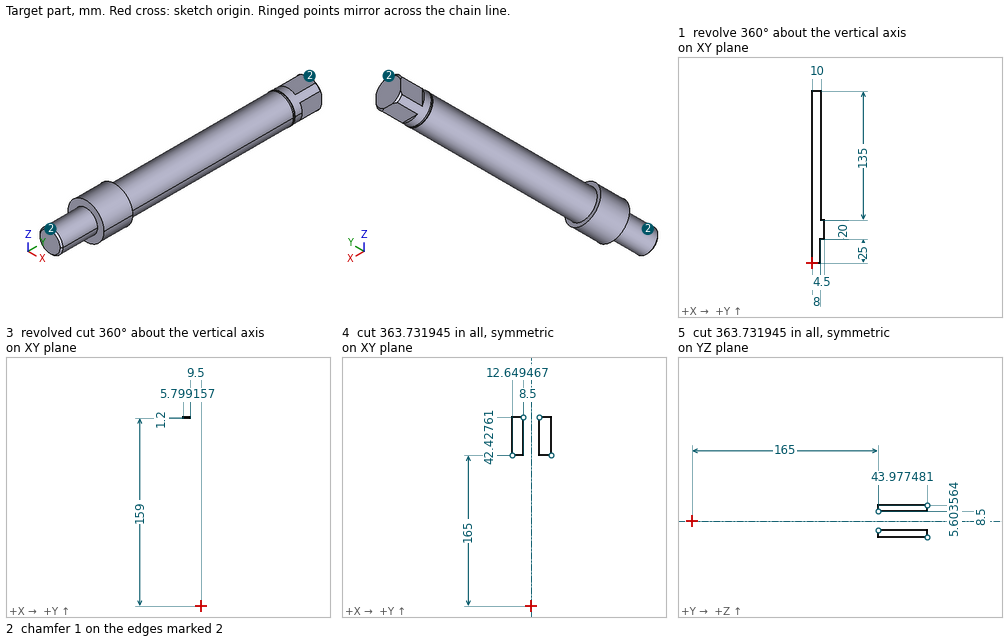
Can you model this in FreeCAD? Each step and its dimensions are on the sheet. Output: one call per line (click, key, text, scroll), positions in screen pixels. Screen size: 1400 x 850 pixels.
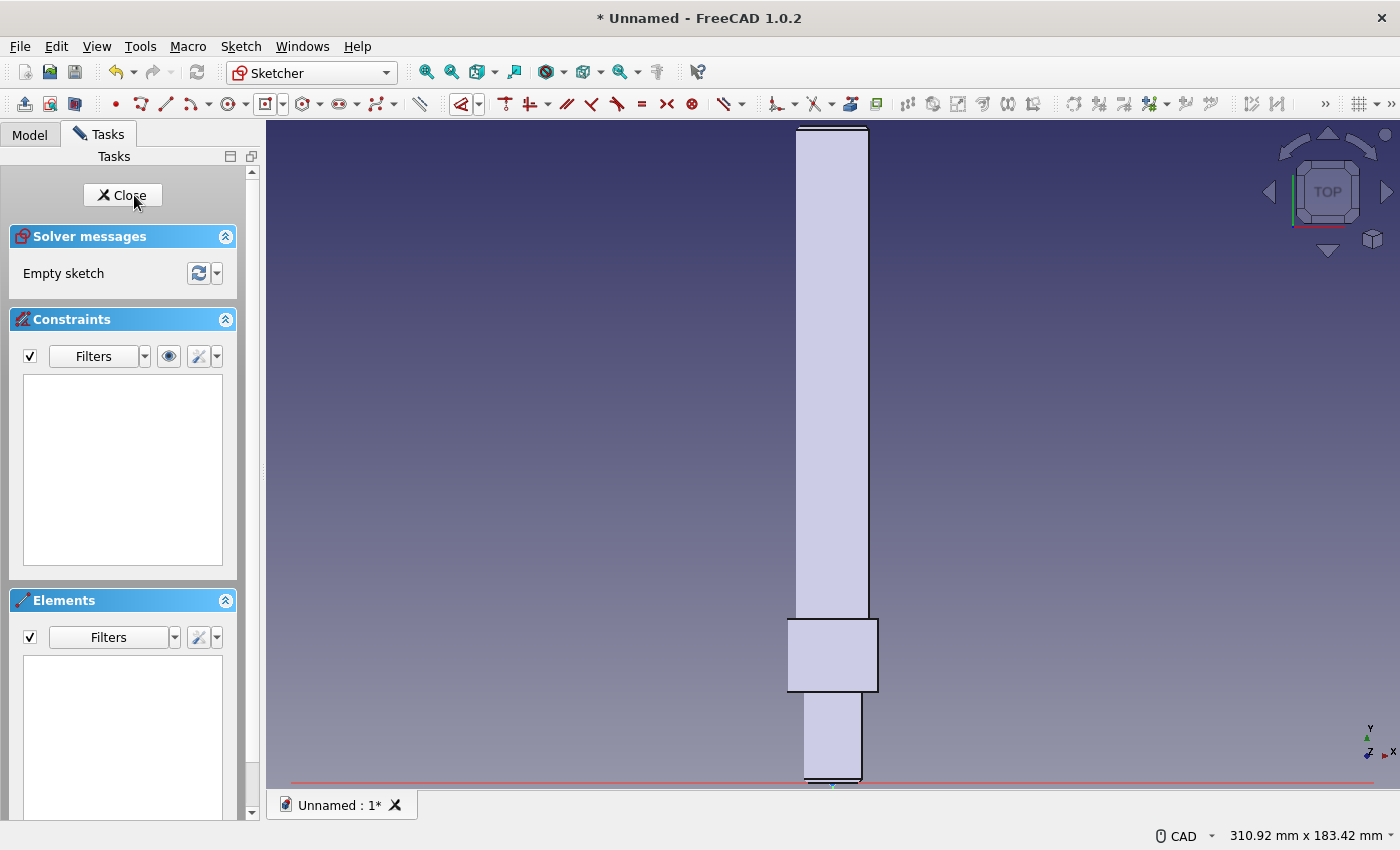
key(q)
key(s)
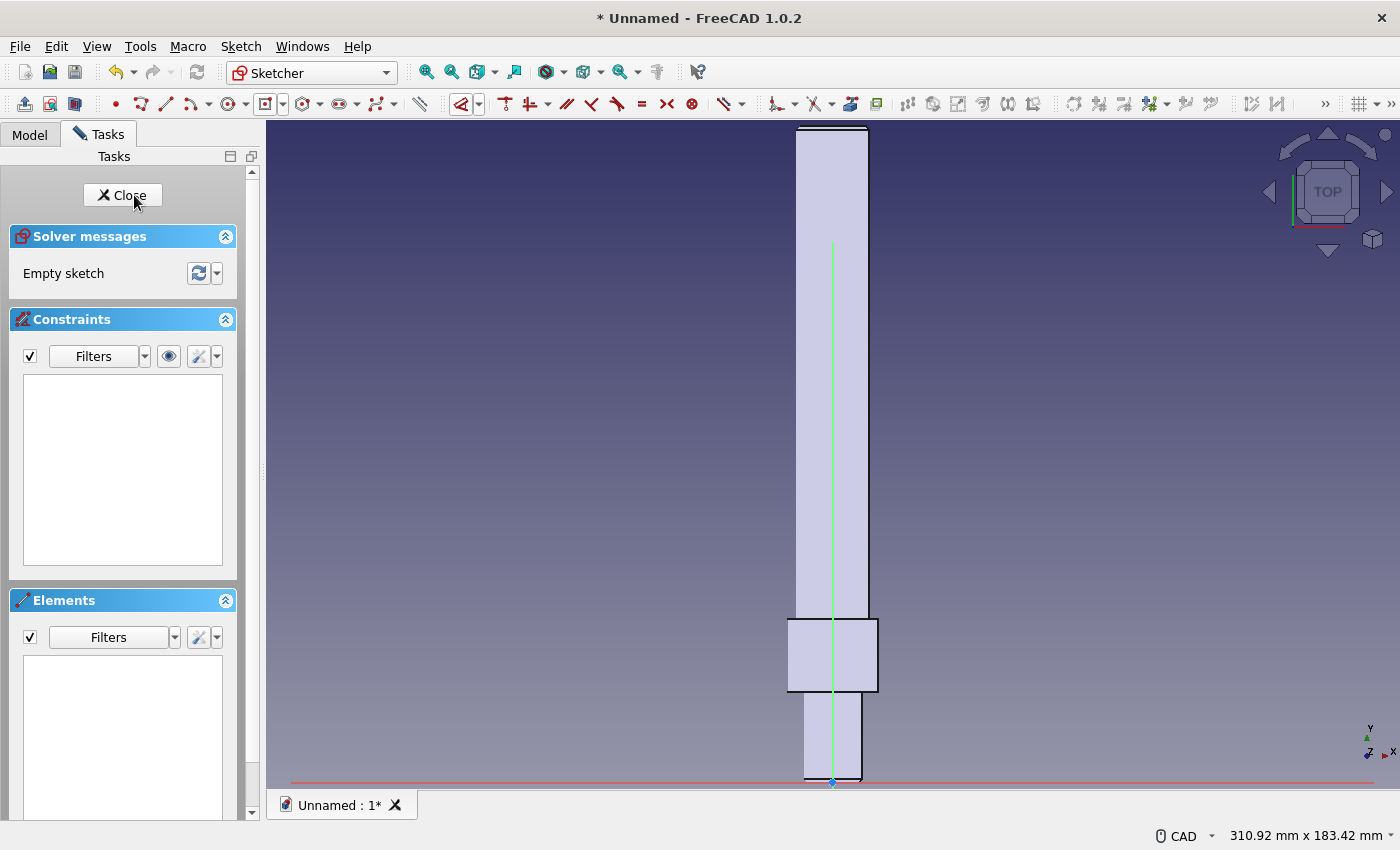
scroll(789, 187, up, 15)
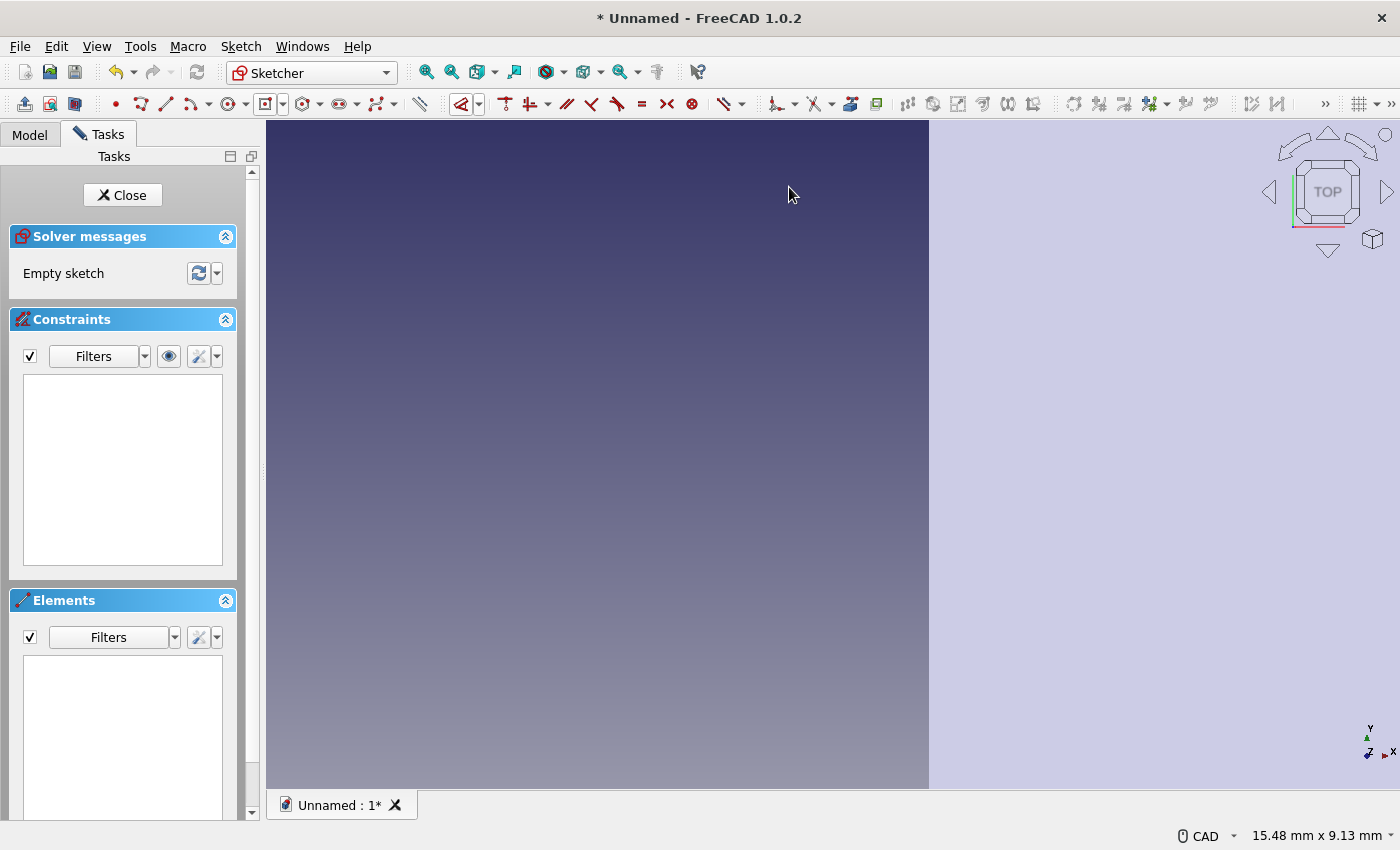
scroll(729, 469, up, 2)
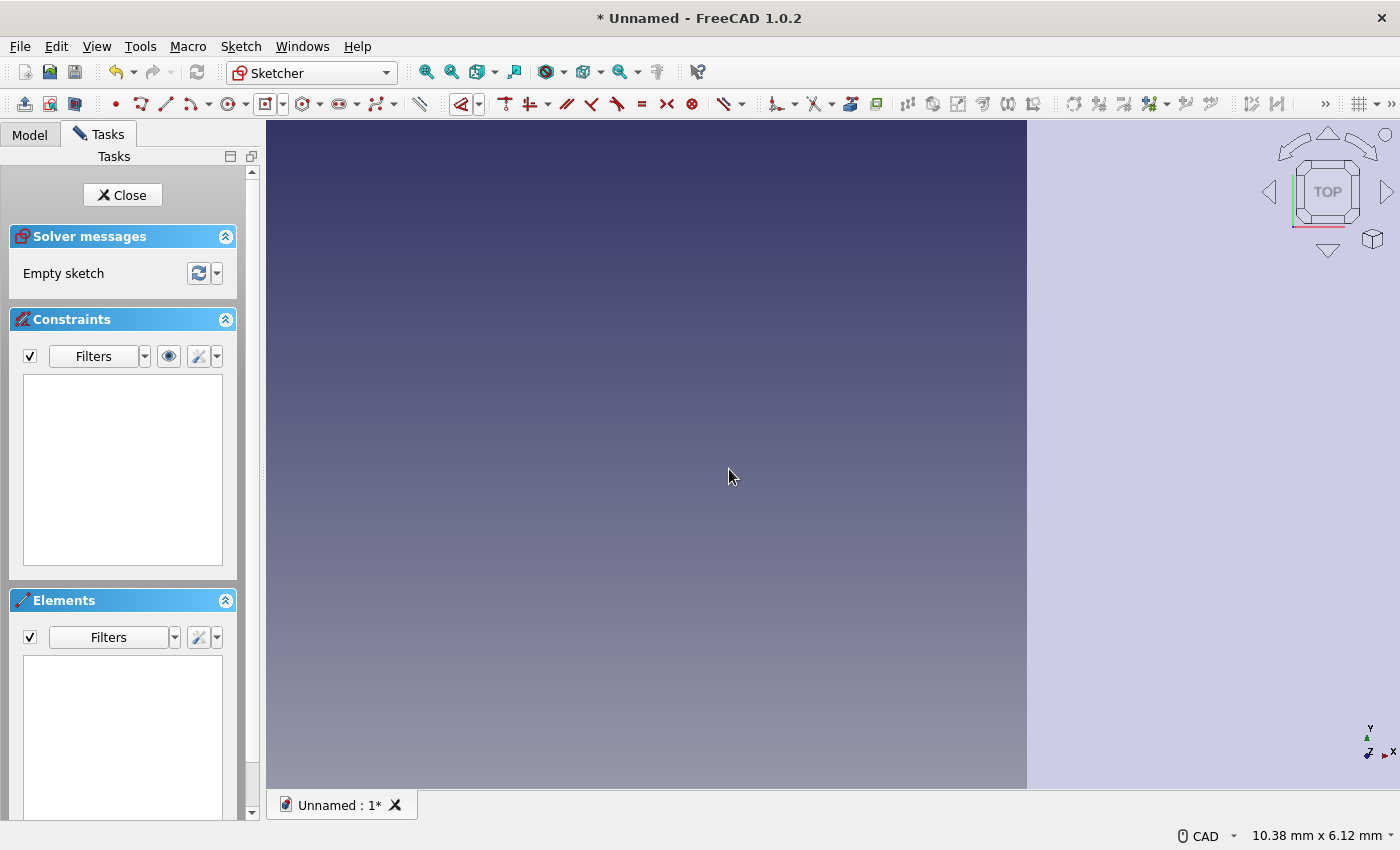
click(282, 104)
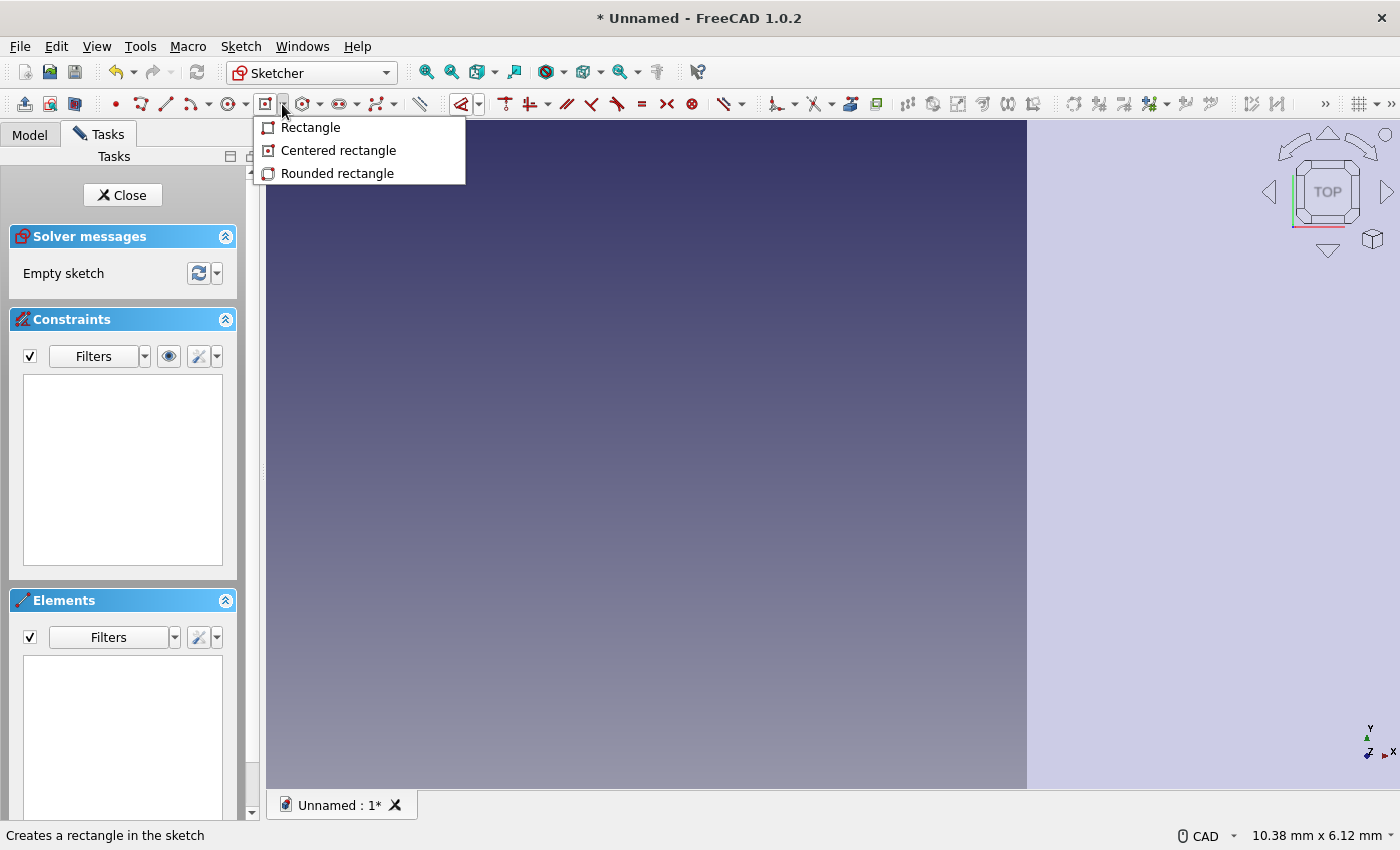
click(360, 128)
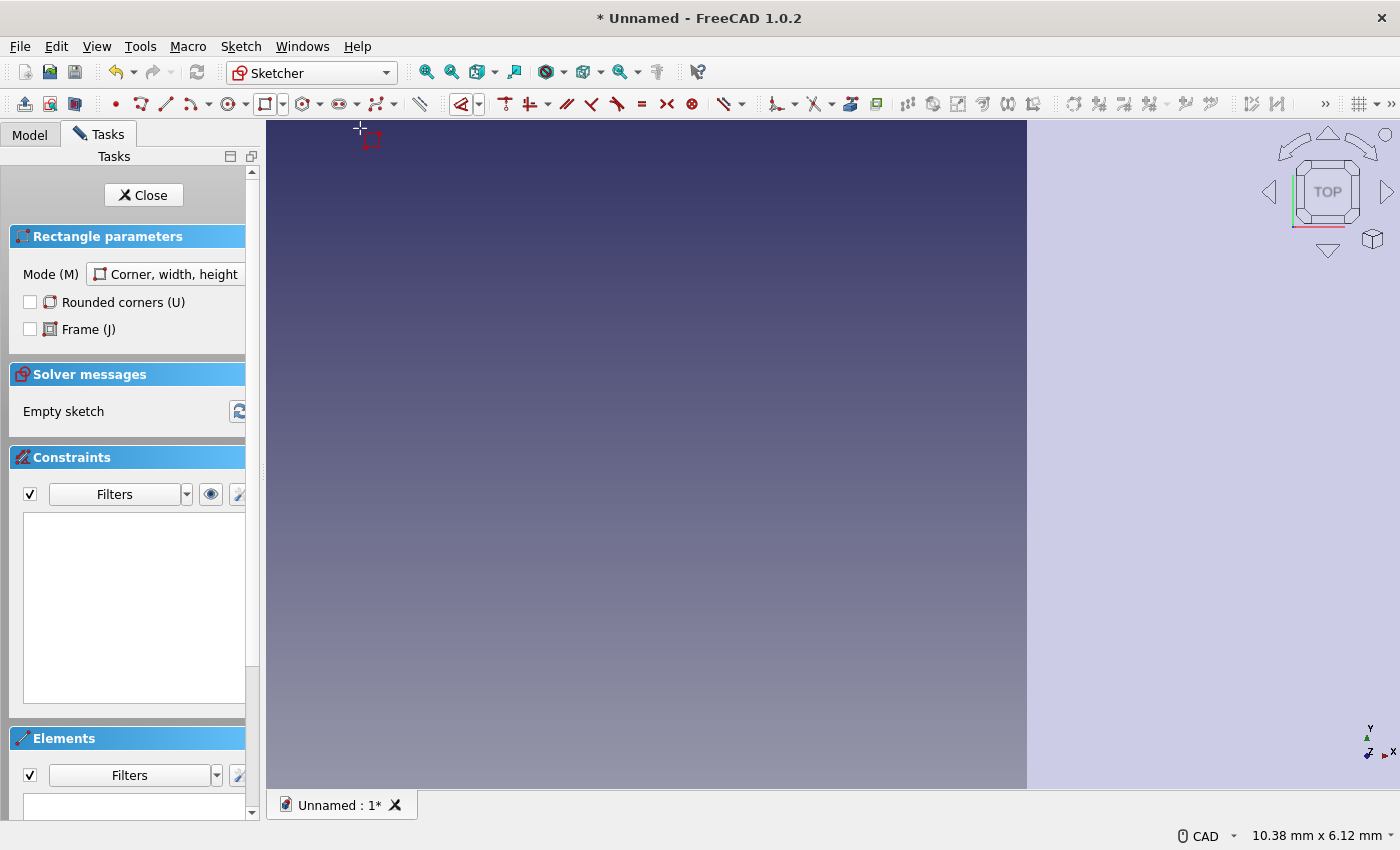
click(448, 389)
click(1081, 520)
key(Escape)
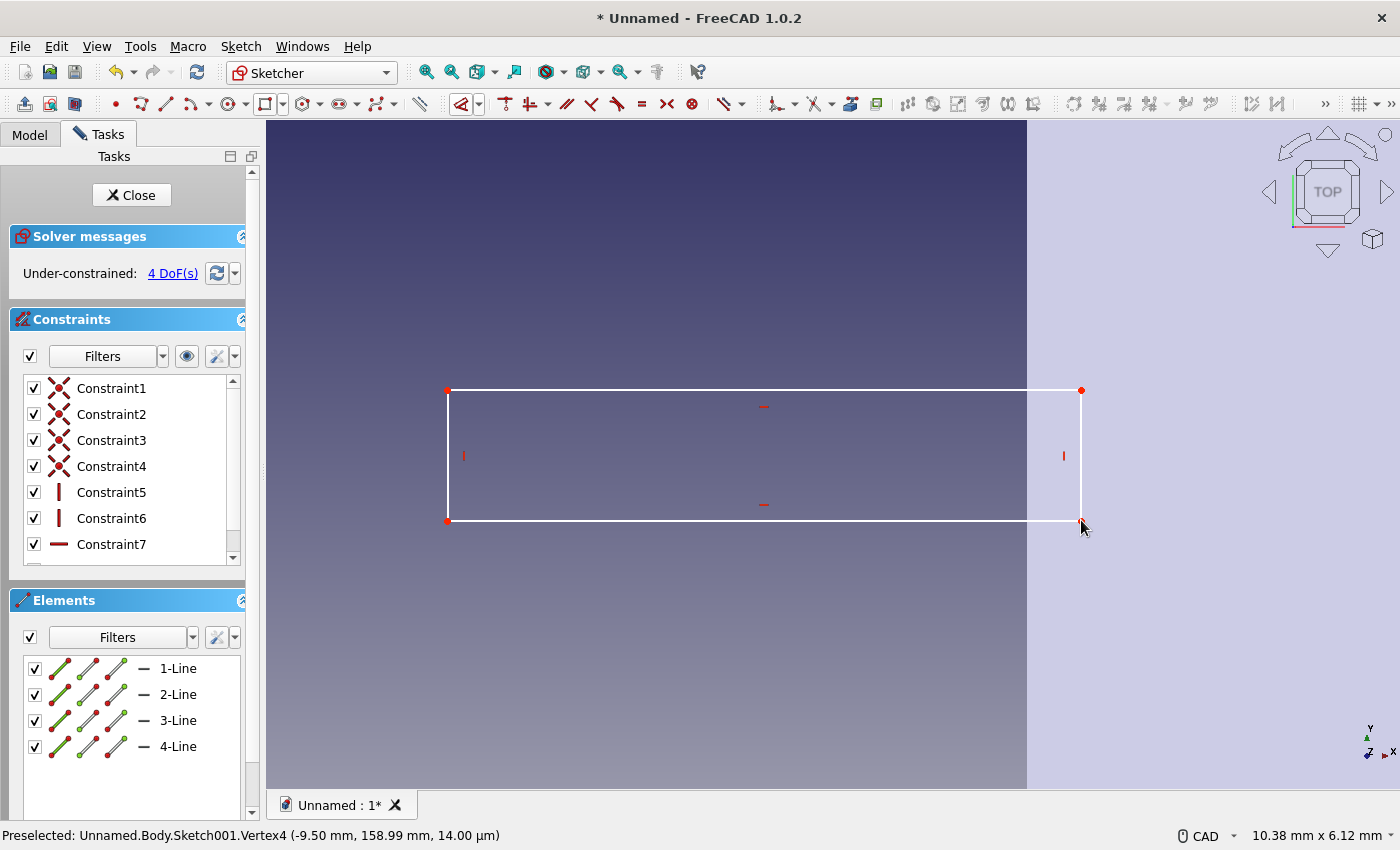
click(460, 104)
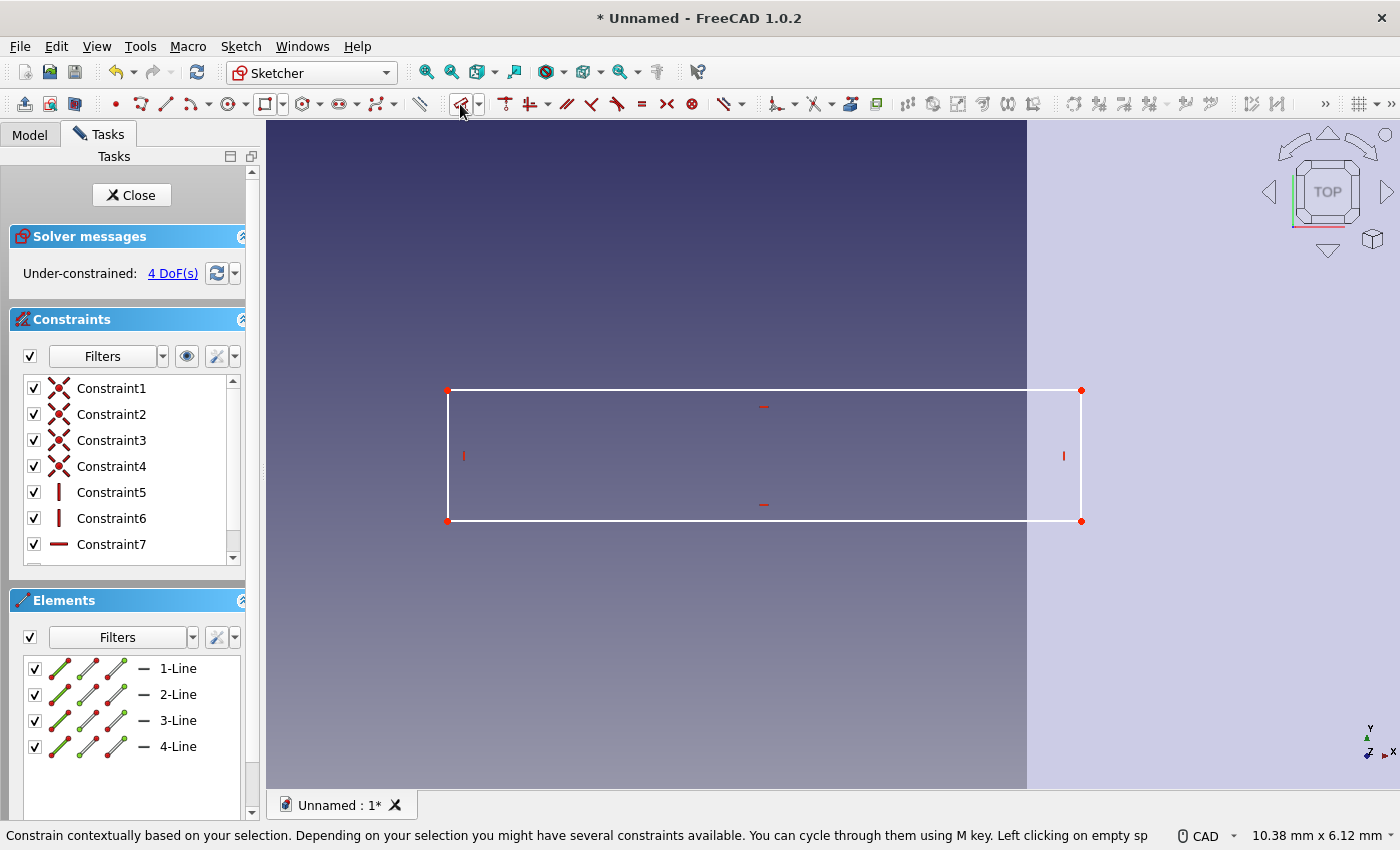
click(448, 429)
click(414, 456)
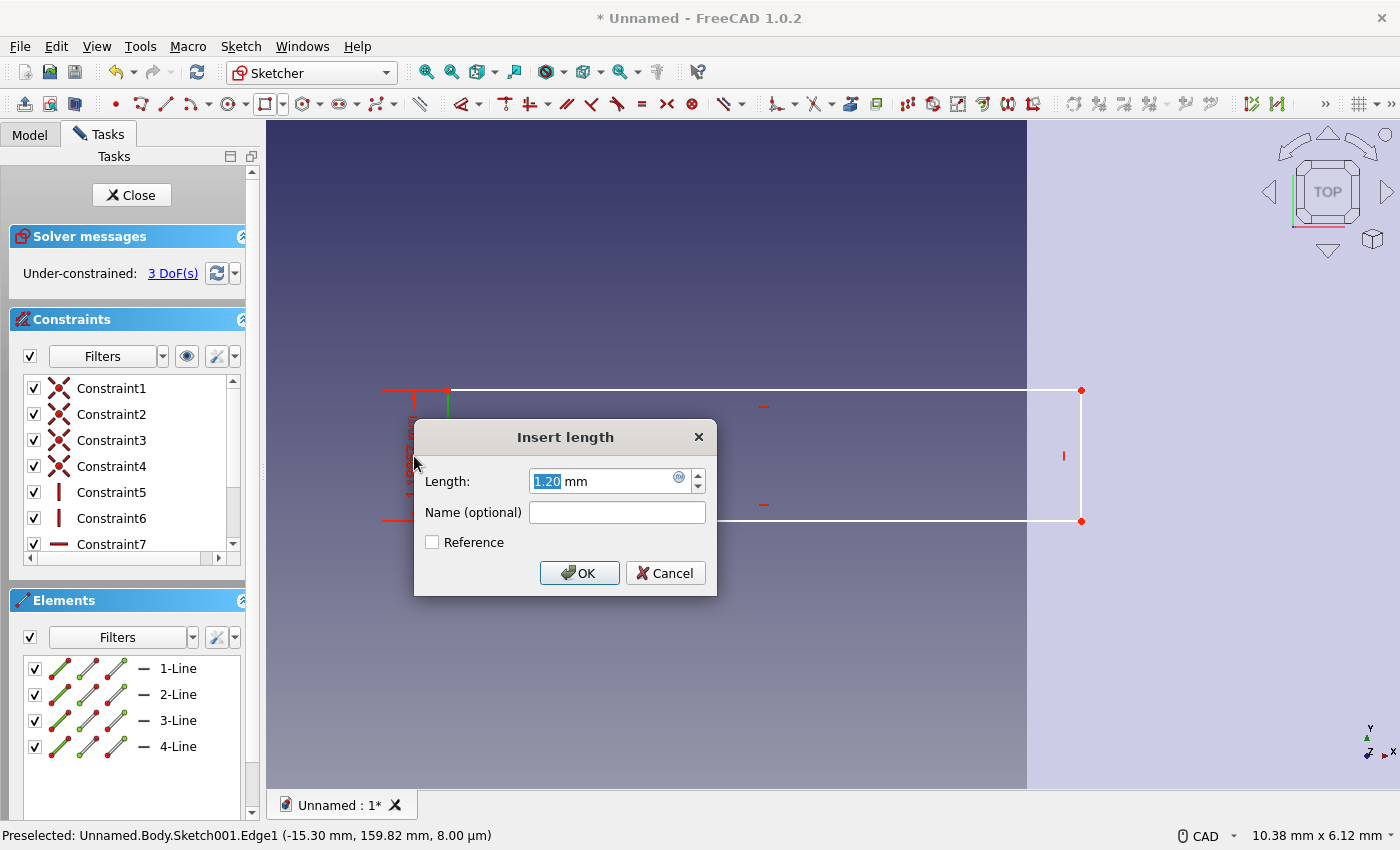
text(1.2)
key(Return)